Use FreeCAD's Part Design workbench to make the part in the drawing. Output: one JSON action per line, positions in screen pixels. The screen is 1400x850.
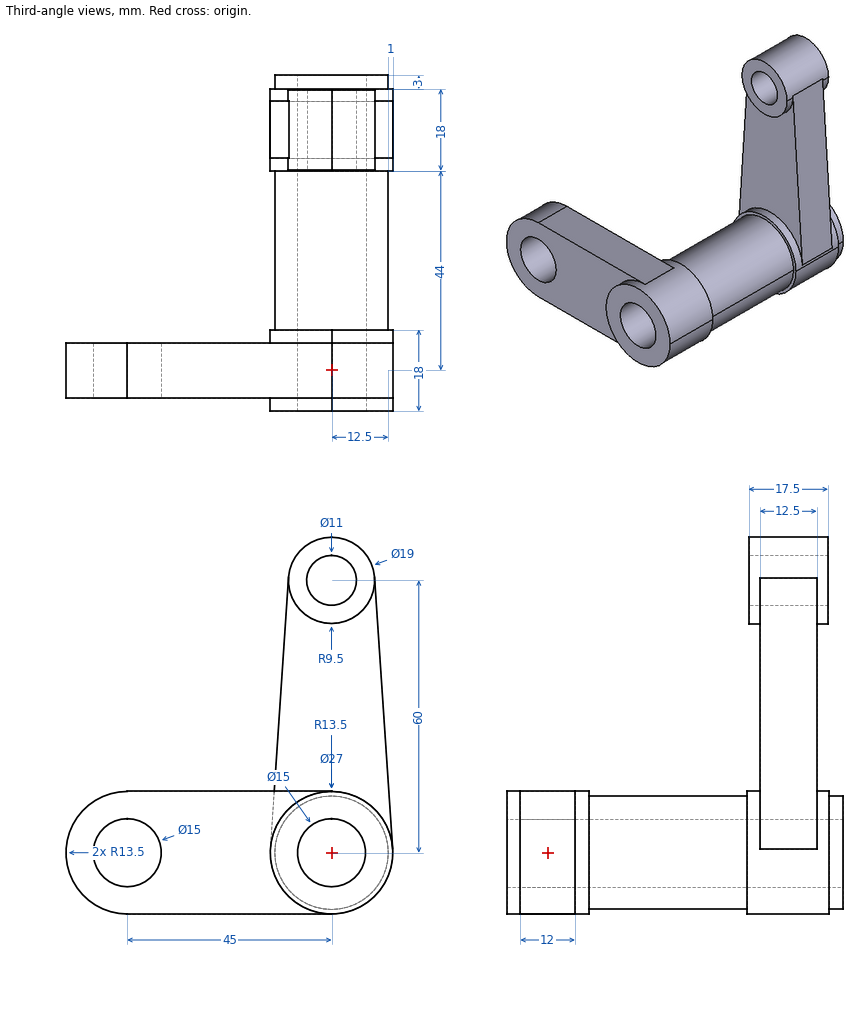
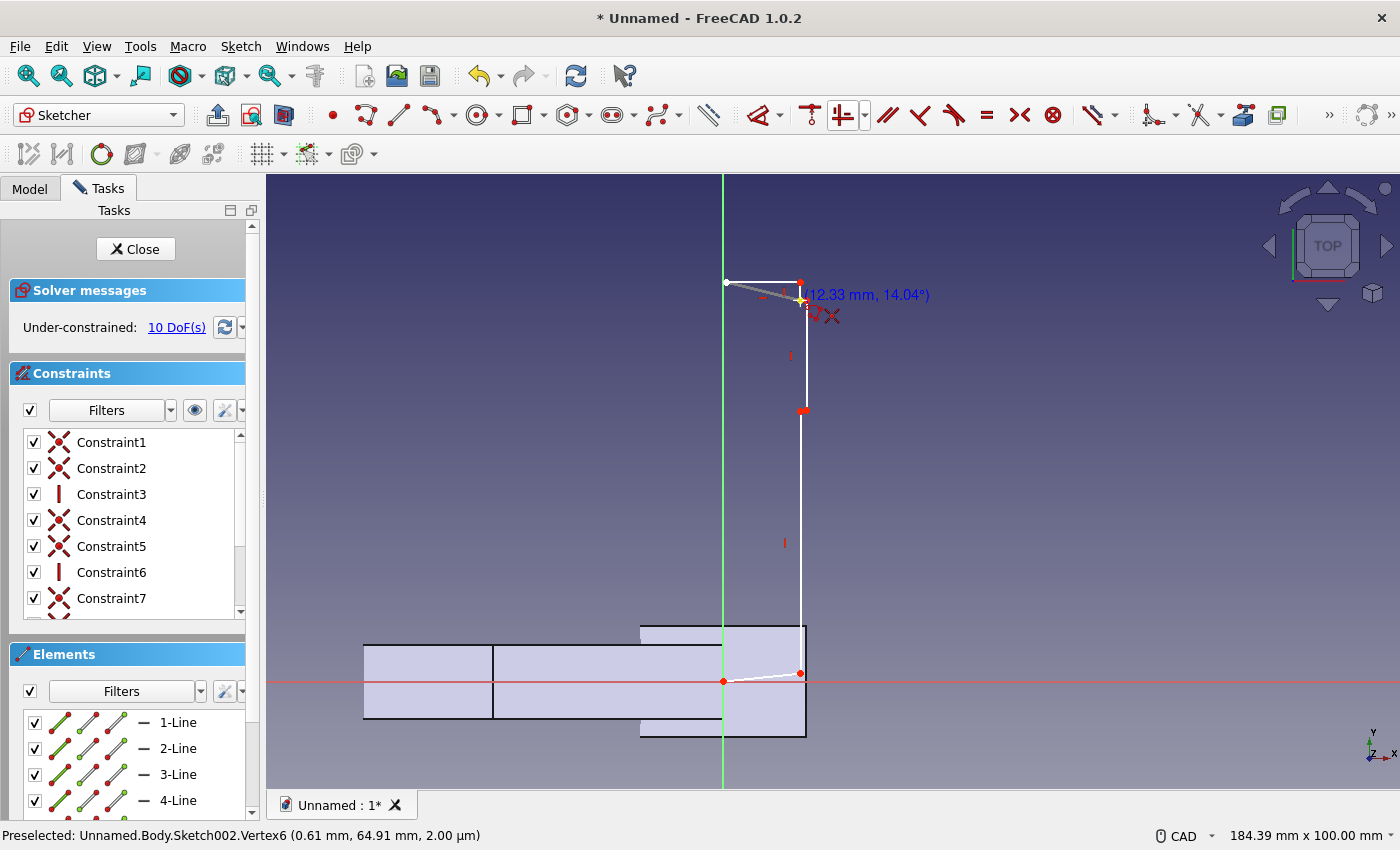
{"action": "left_click", "coordinate": [723, 682]}
{"action": "key", "text": "Escape"}
{"action": "key", "text": "Escape"}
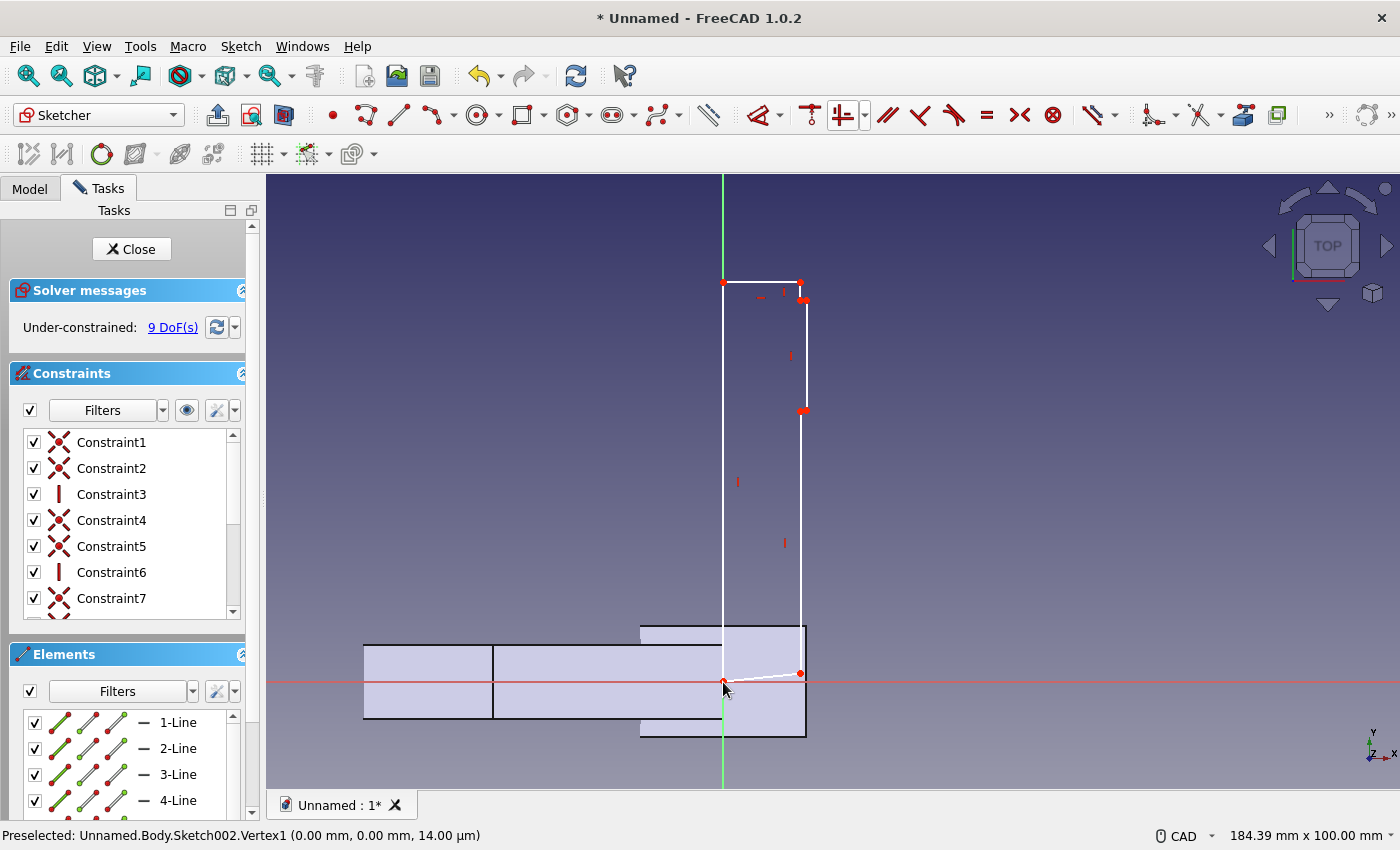
{"action": "left_click", "coordinate": [747, 679]}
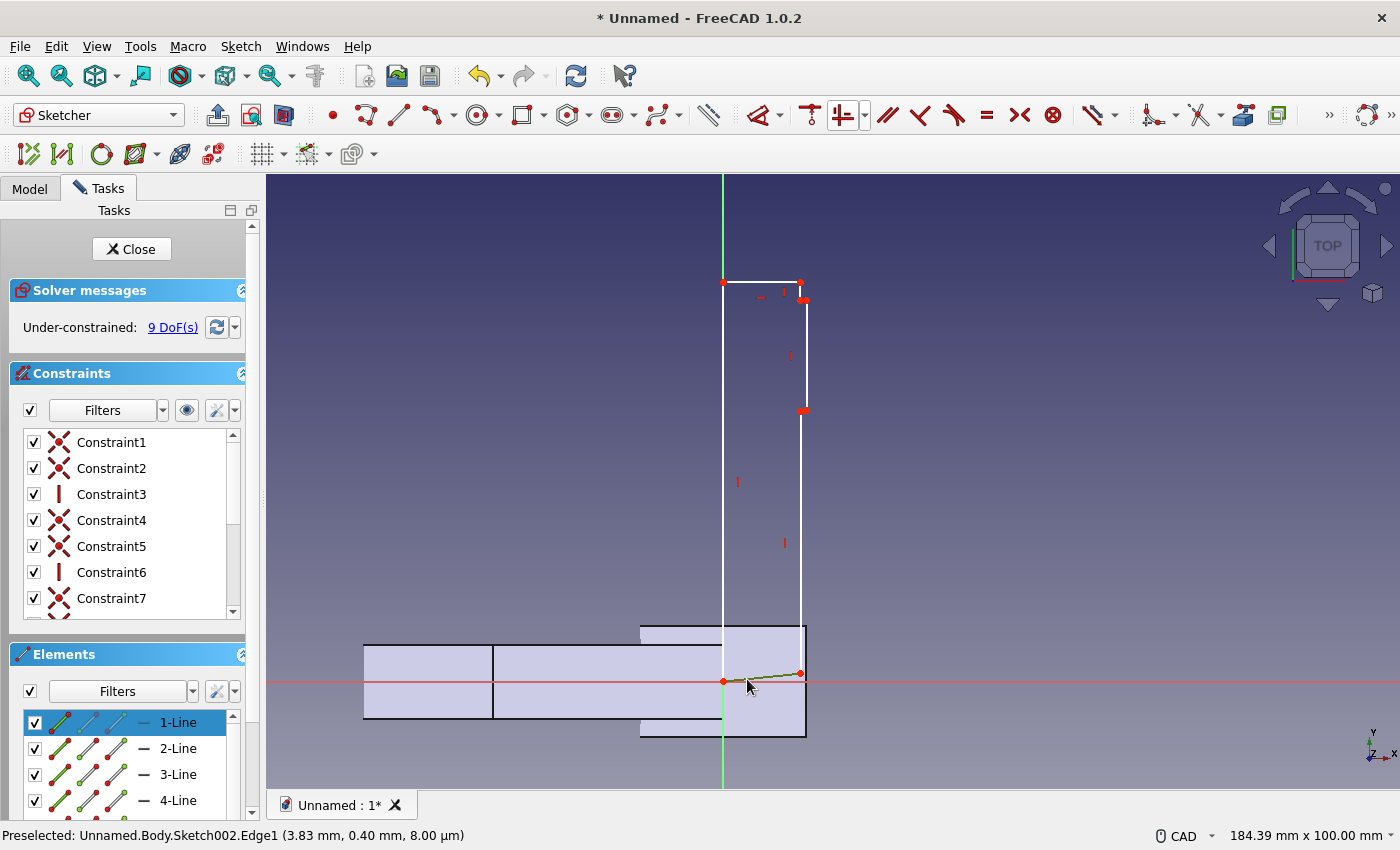
{"action": "key", "text": "h"}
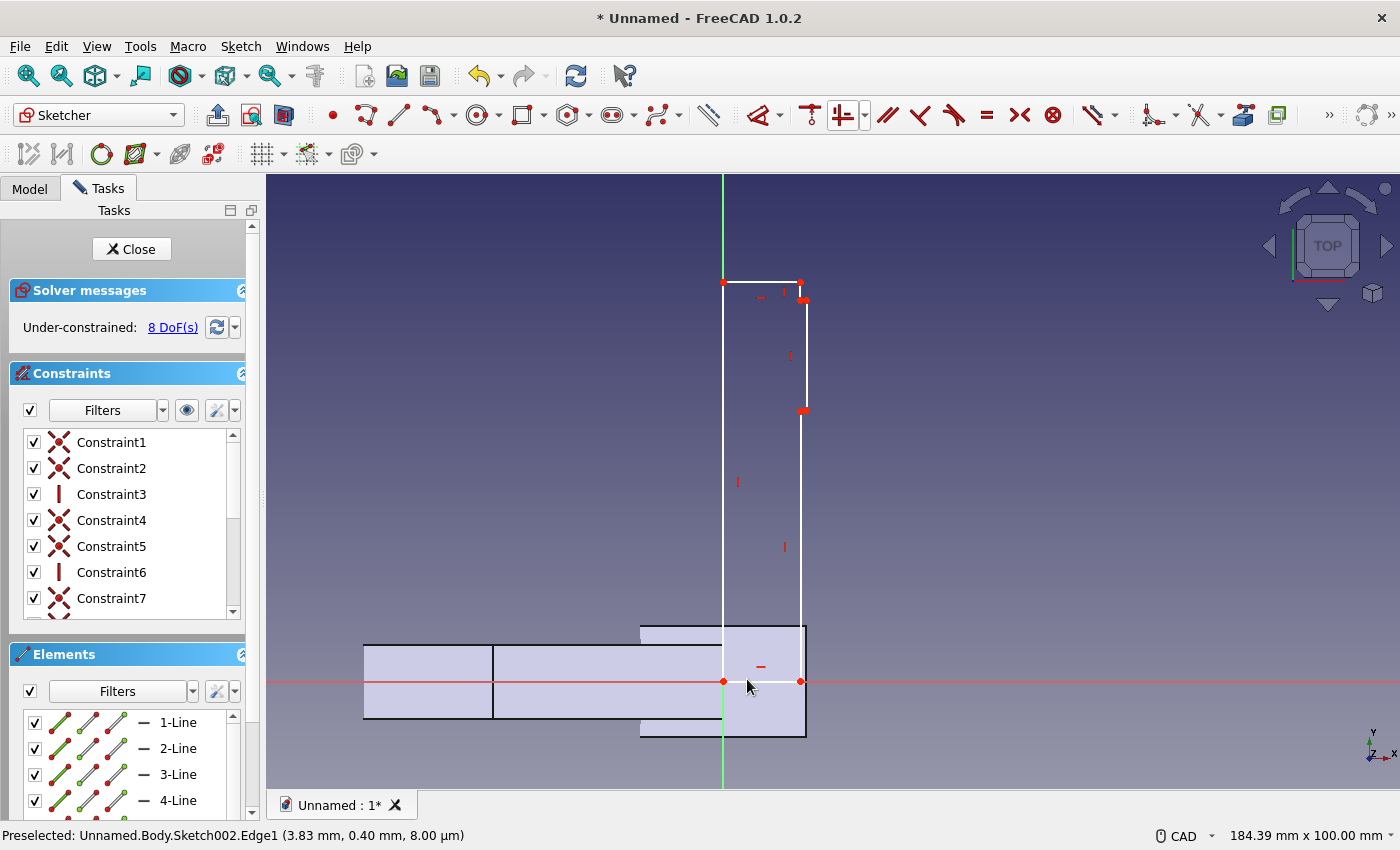
{"action": "scroll", "coordinate": [804, 411], "scroll_direction": "up", "scroll_amount": 8}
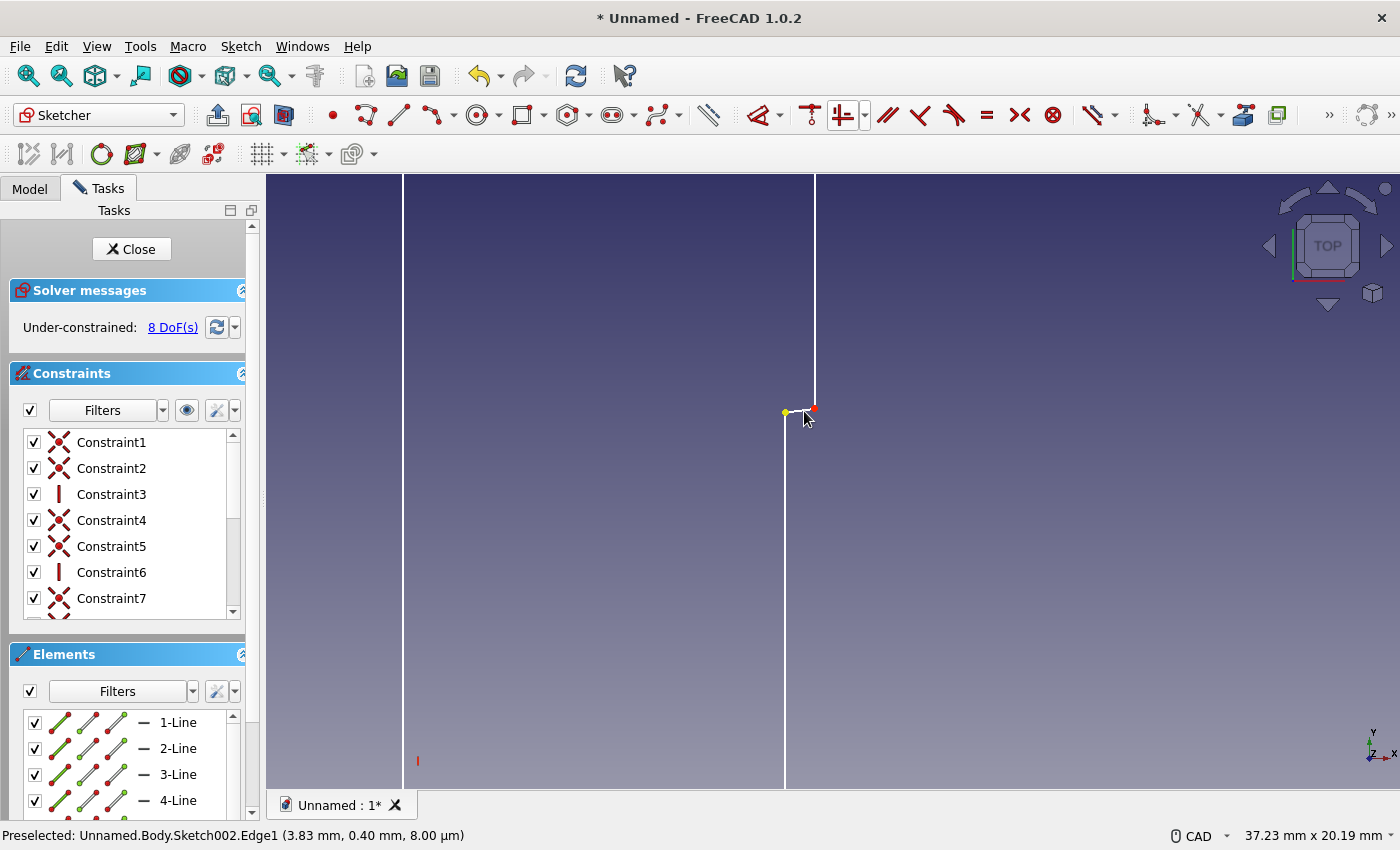
{"action": "left_click", "coordinate": [800, 411]}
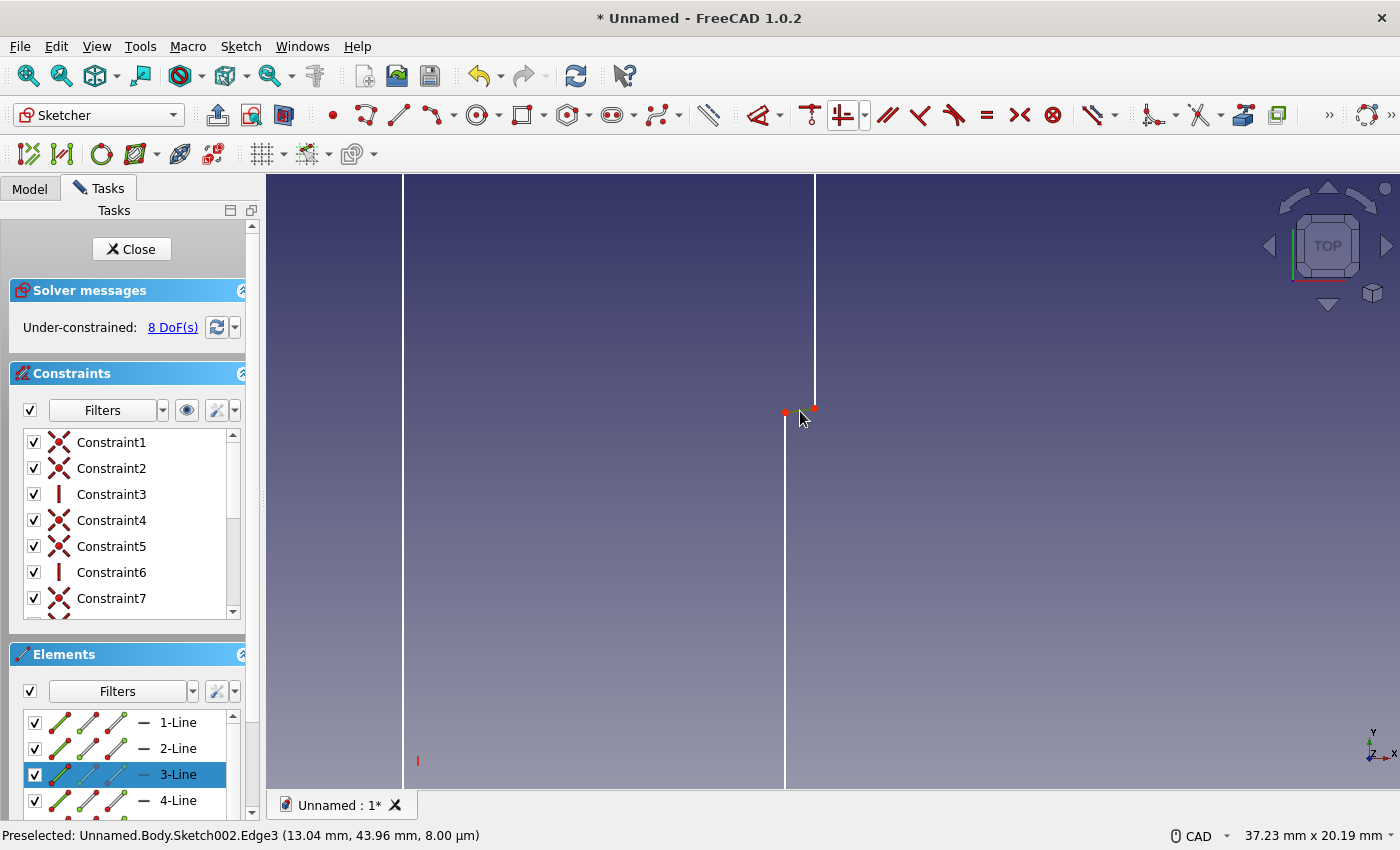
{"action": "key", "text": "h"}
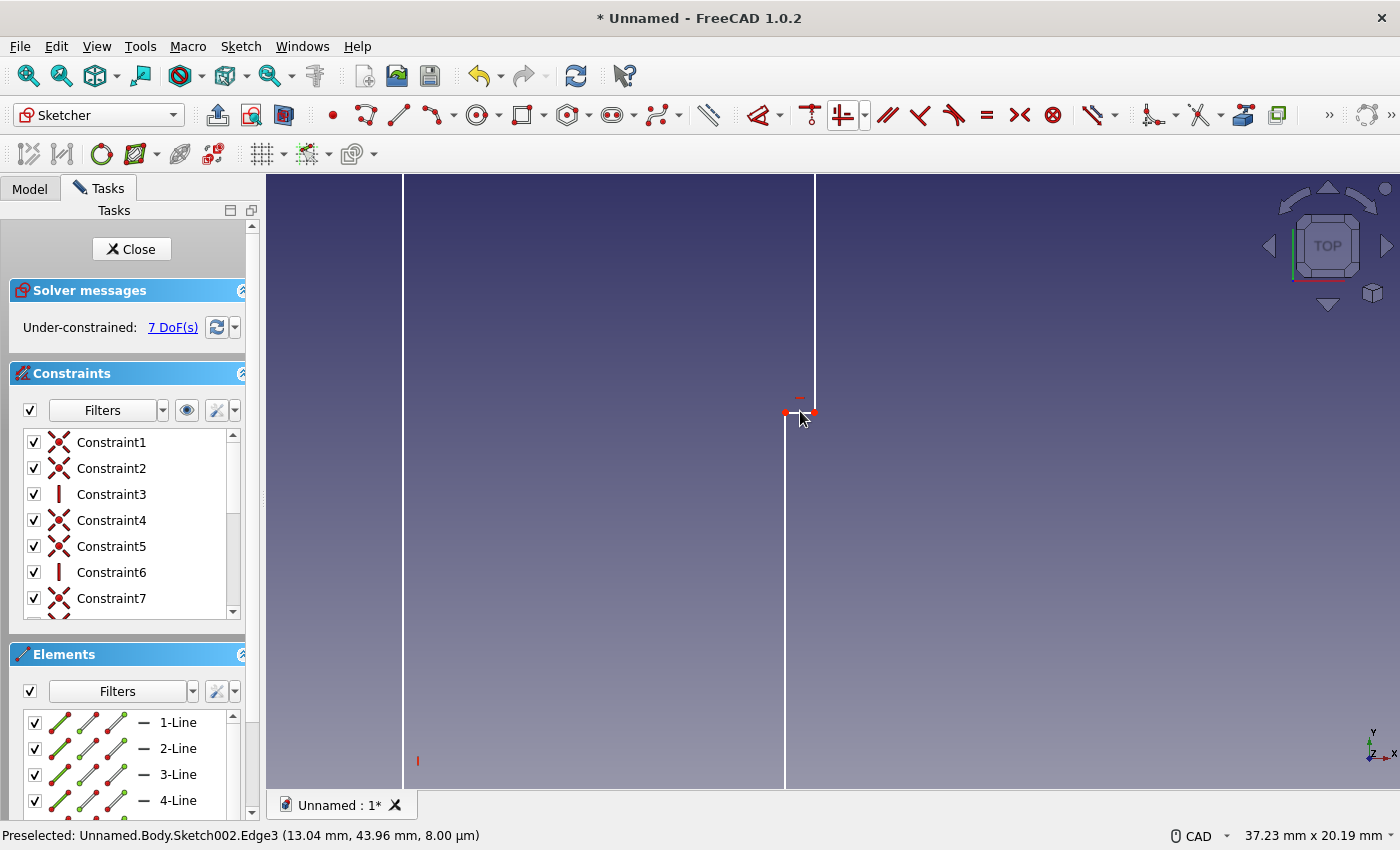
{"action": "scroll", "coordinate": [804, 411], "scroll_direction": "down", "scroll_amount": 8}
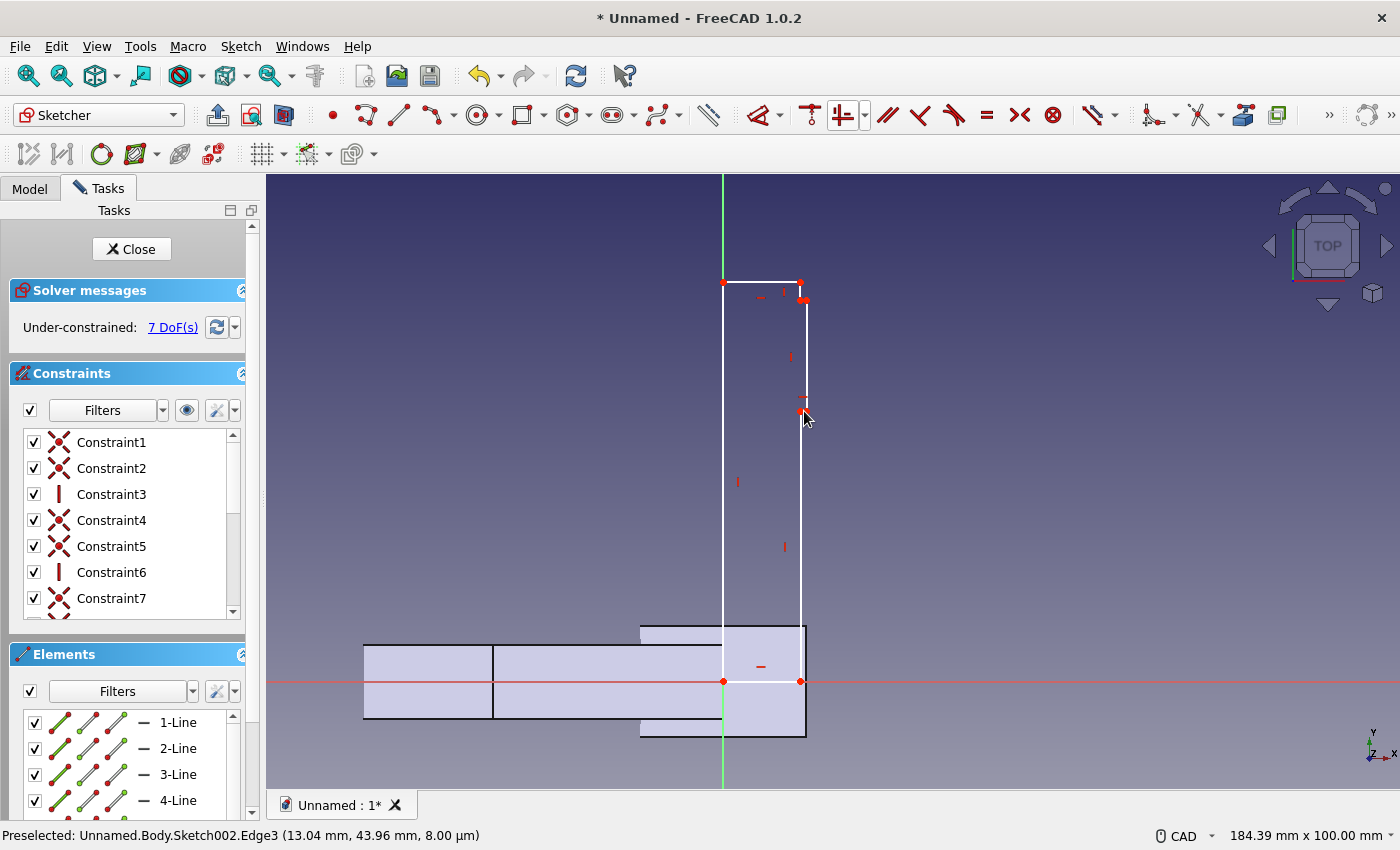
{"action": "scroll", "coordinate": [805, 301], "scroll_direction": "up", "scroll_amount": 10}